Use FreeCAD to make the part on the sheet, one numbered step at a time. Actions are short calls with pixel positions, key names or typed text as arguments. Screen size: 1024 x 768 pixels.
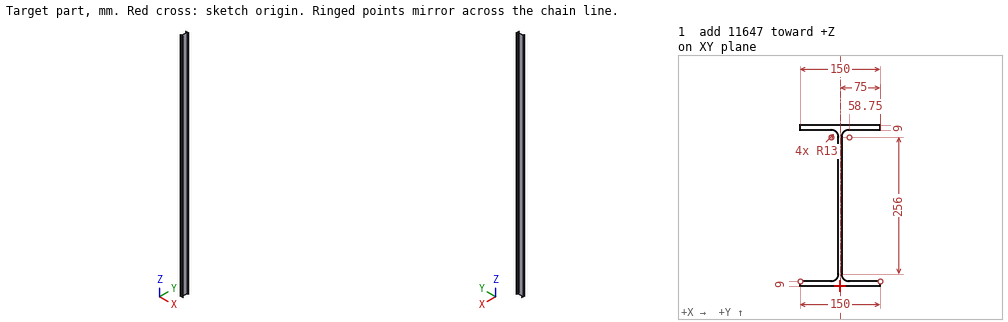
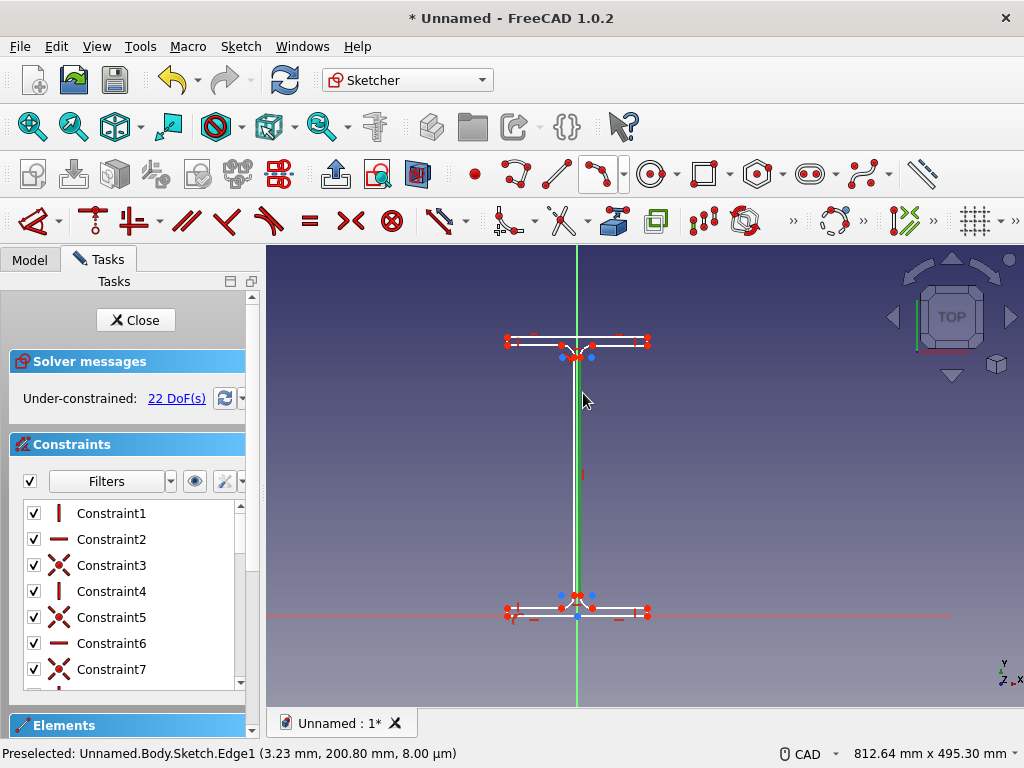
scroll(582, 601, up, 6)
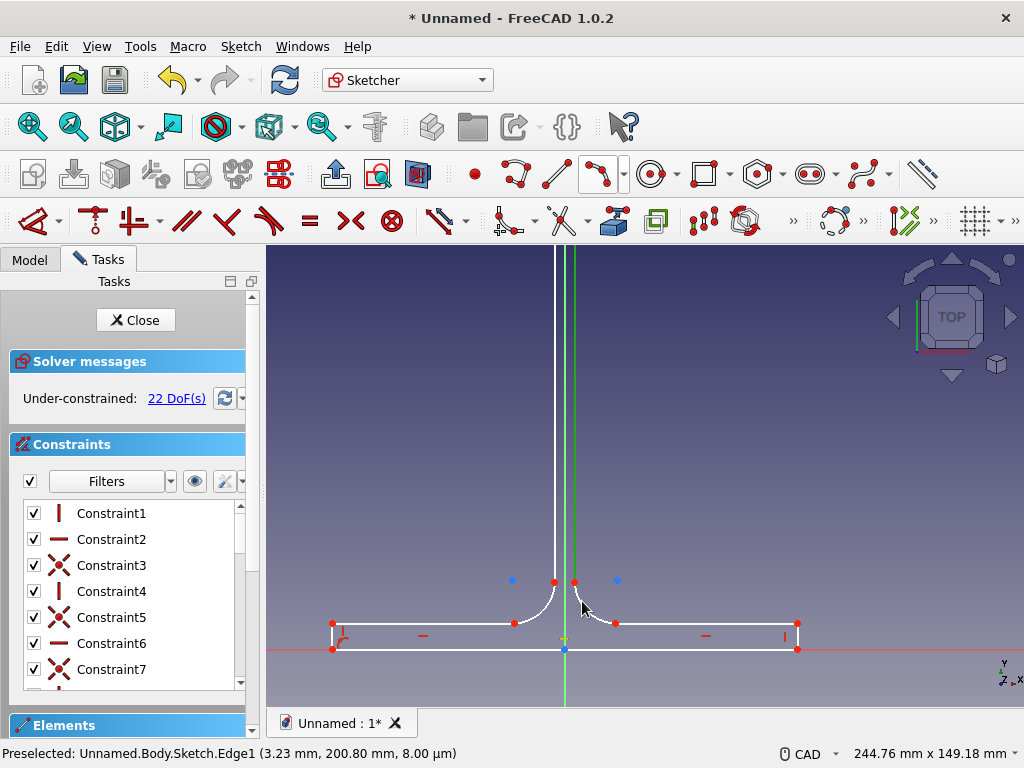
click(580, 601)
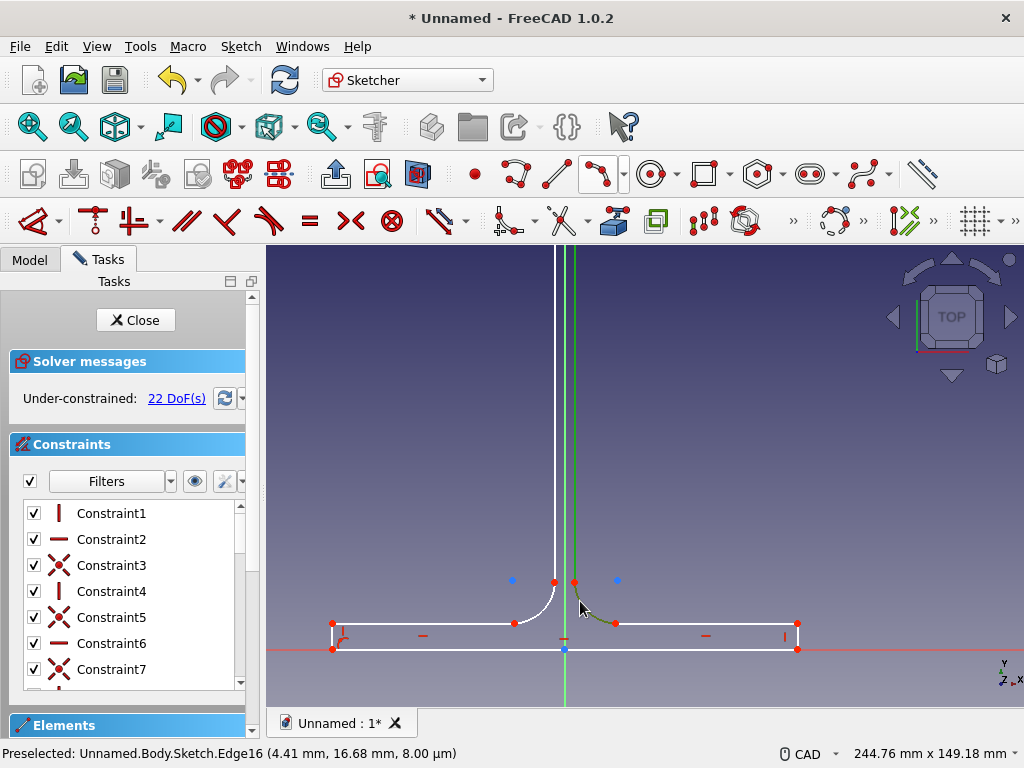
key(t)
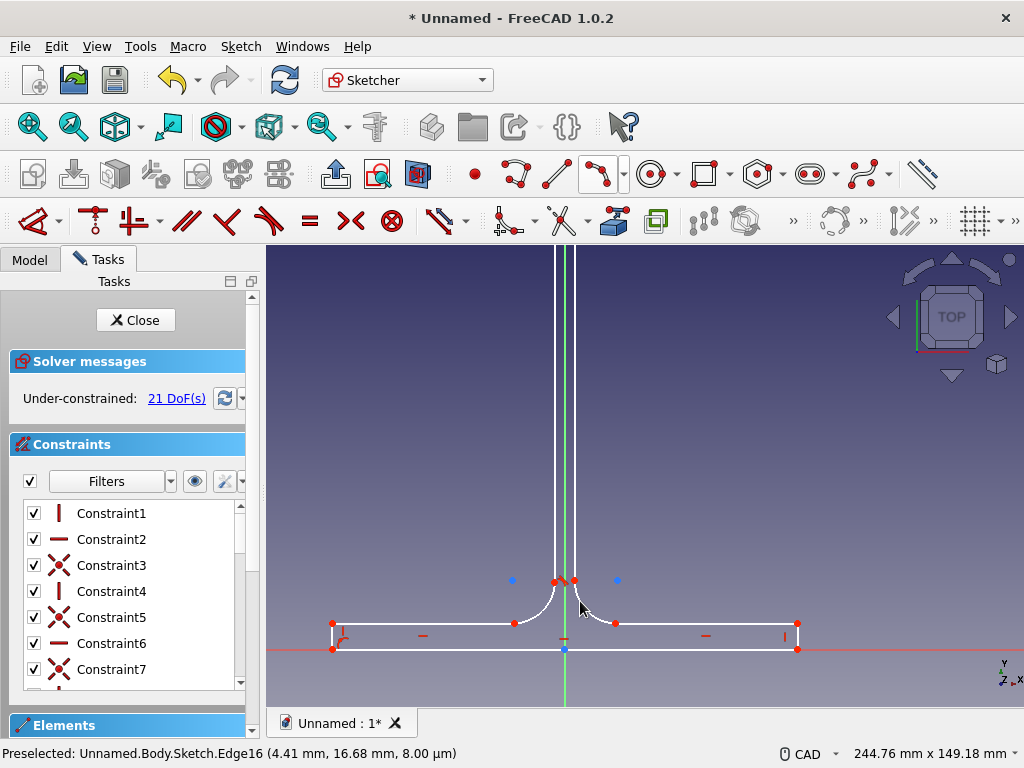
scroll(582, 601, down, 6)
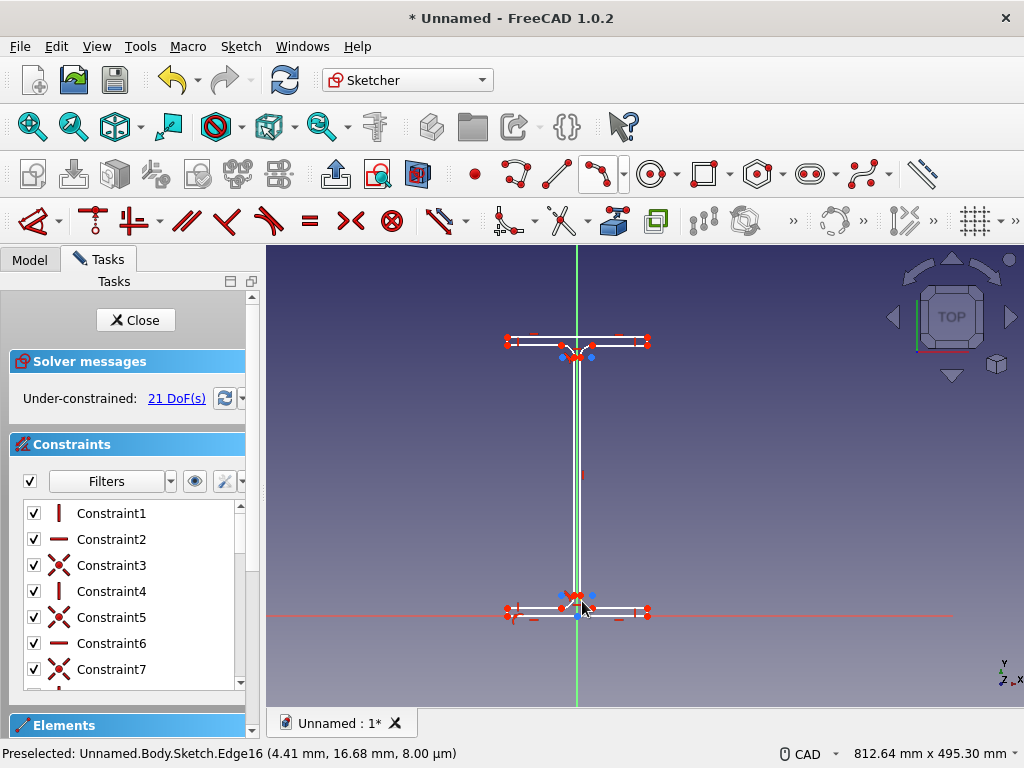
scroll(609, 346, up, 3)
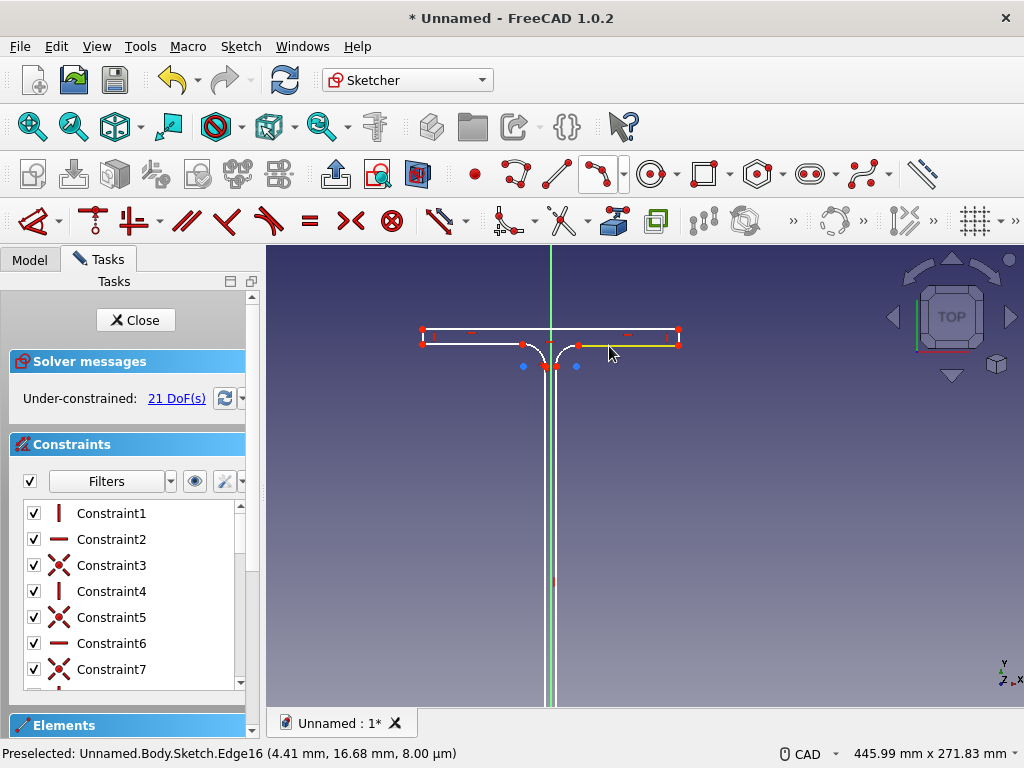
click(609, 346)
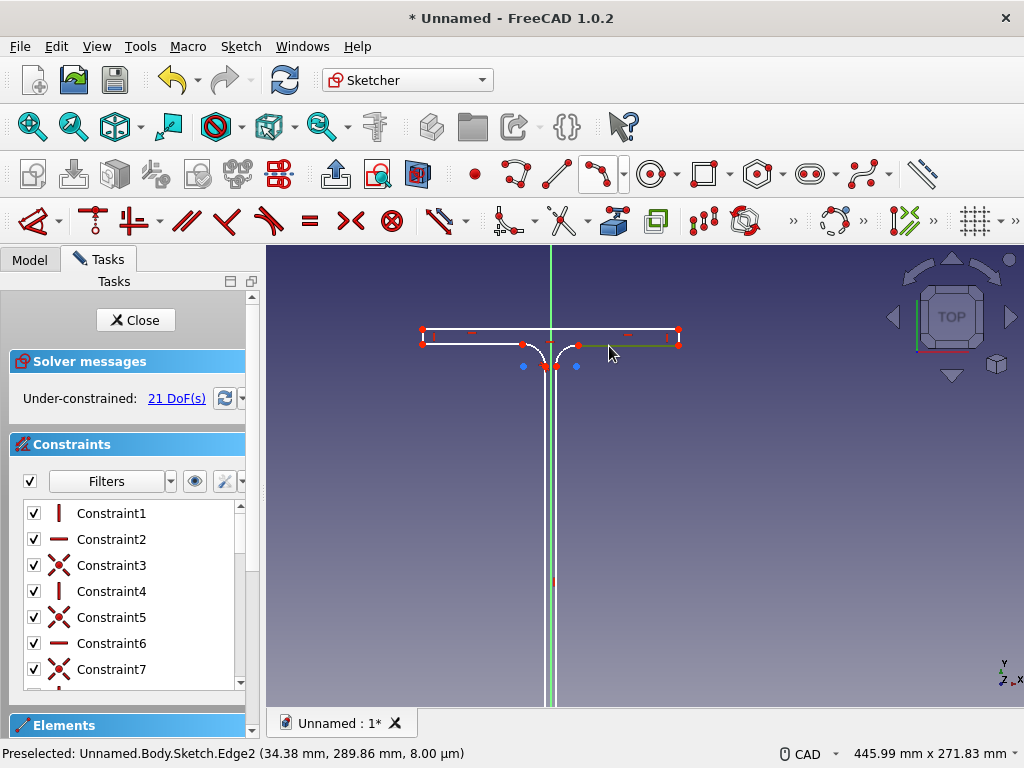
scroll(568, 347, up, 2)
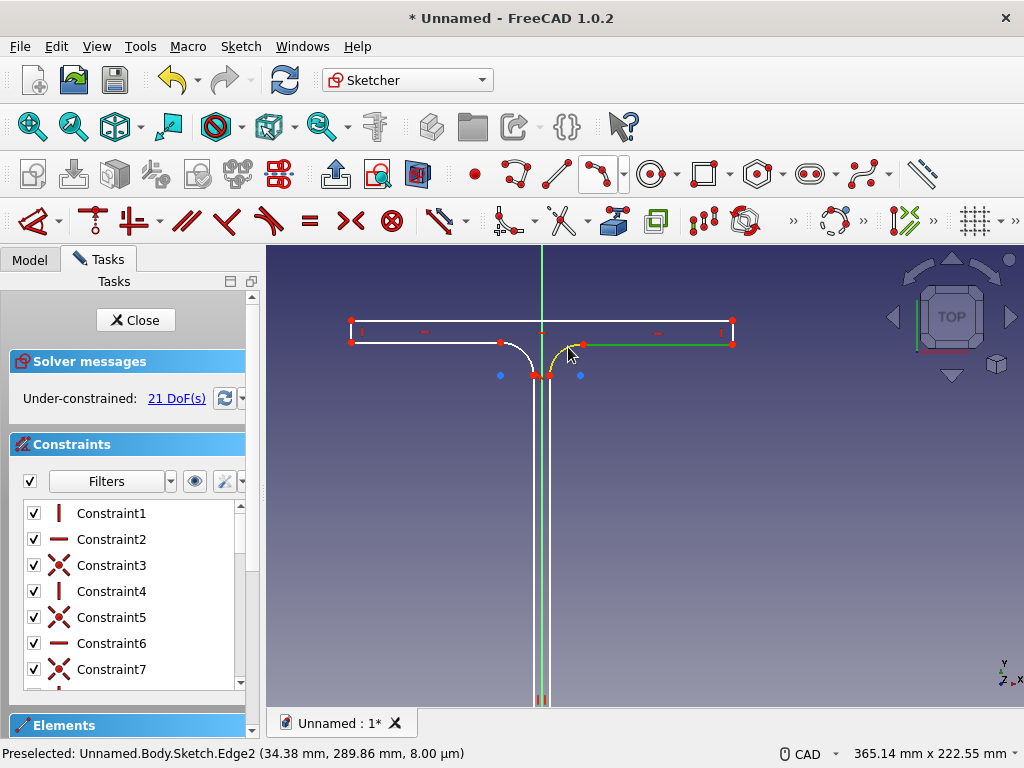
click(569, 347)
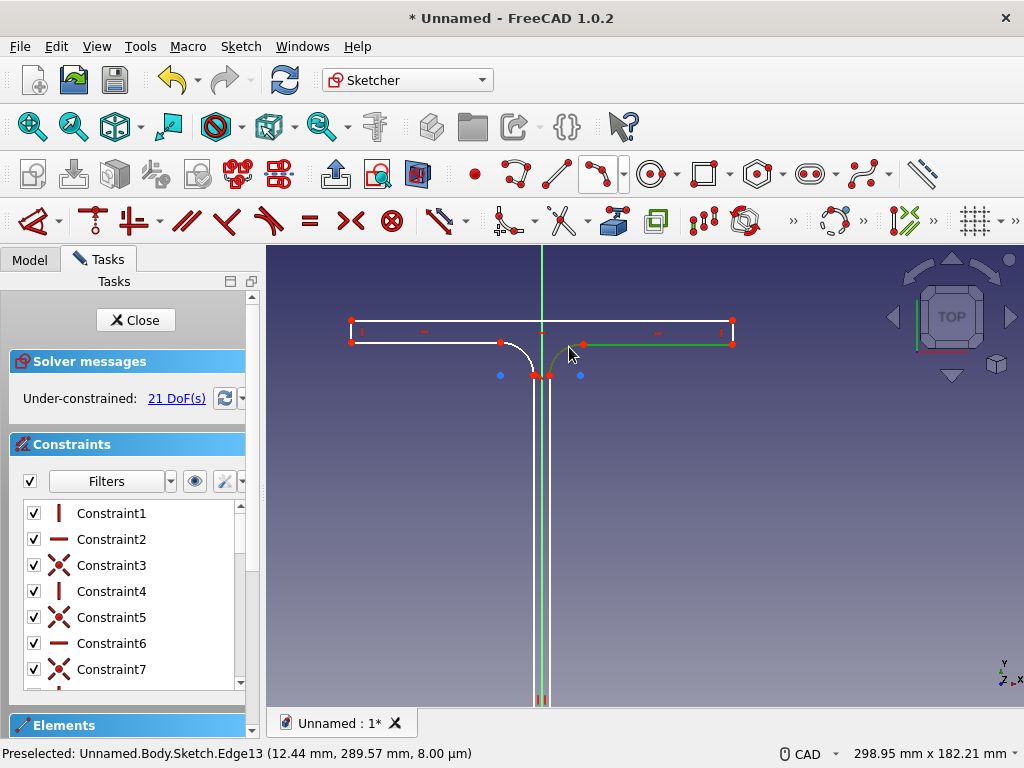
key(t)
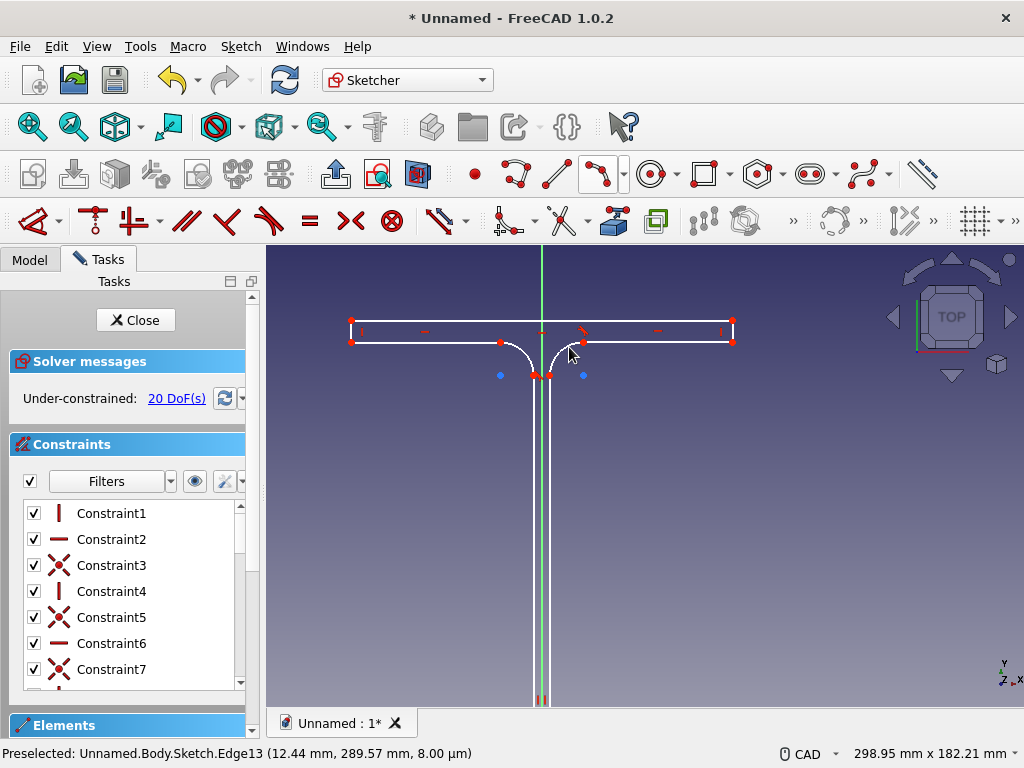
click(396, 343)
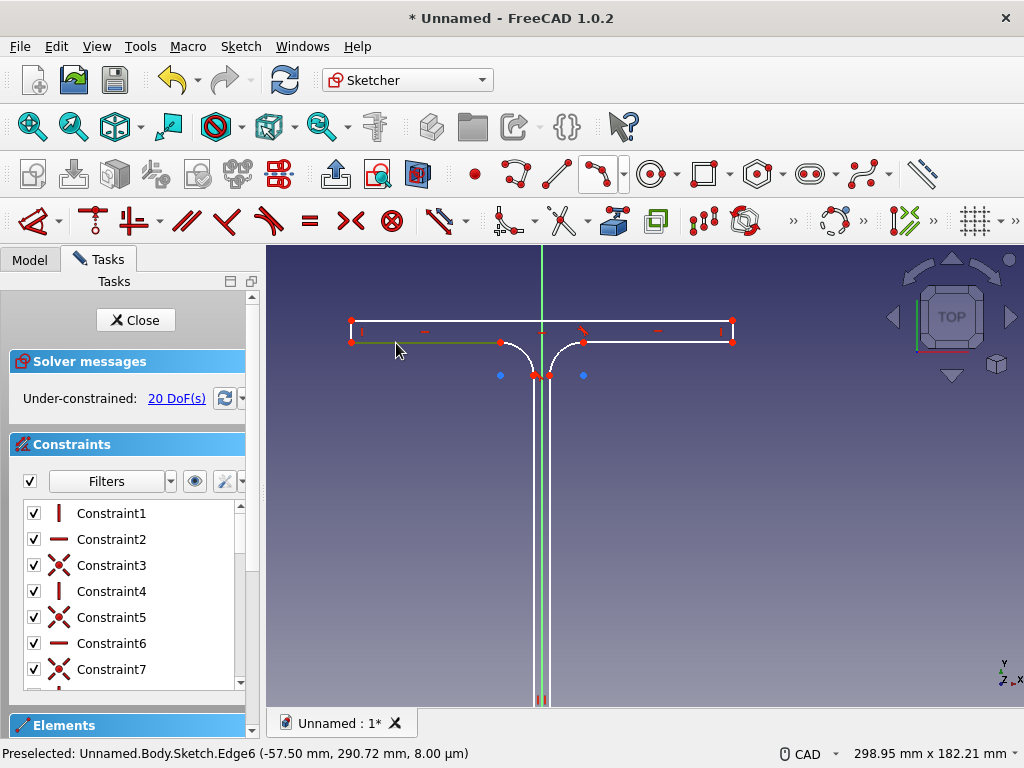
click(530, 361)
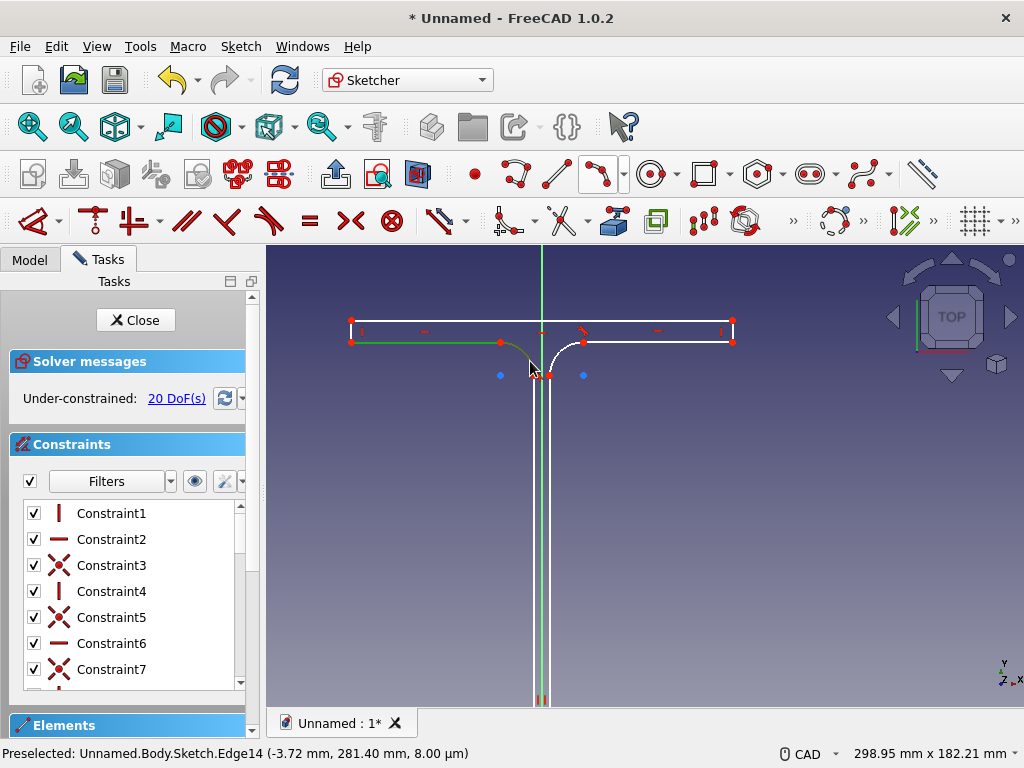
key(t)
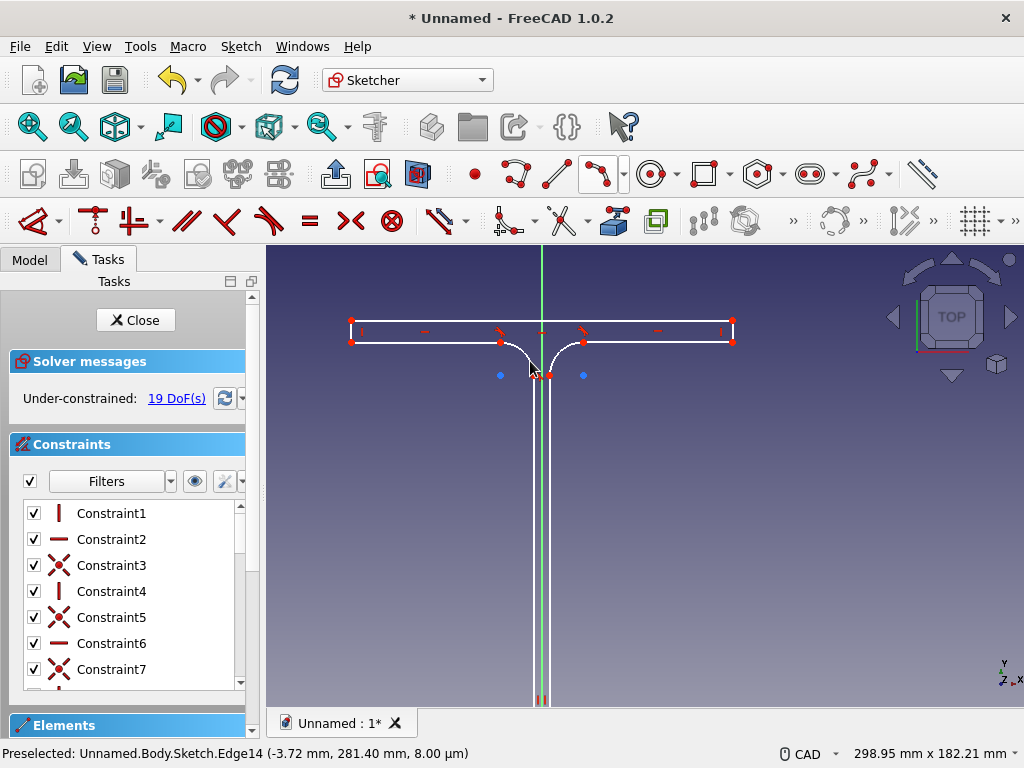
scroll(534, 570, up, 3)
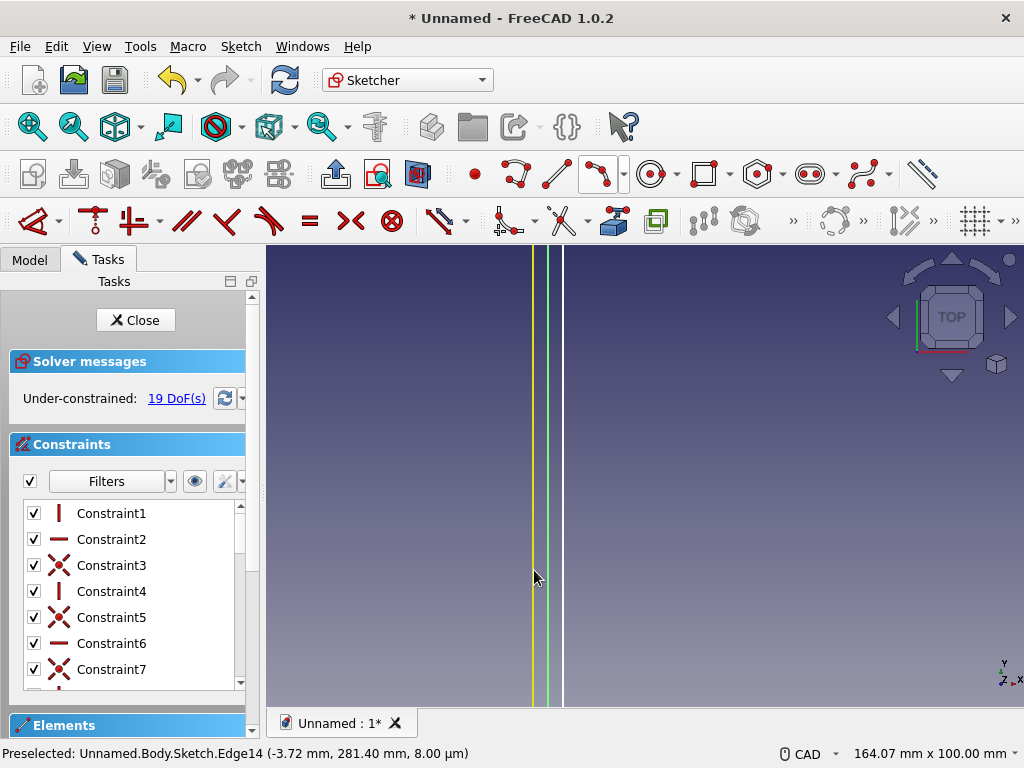
click(533, 570)